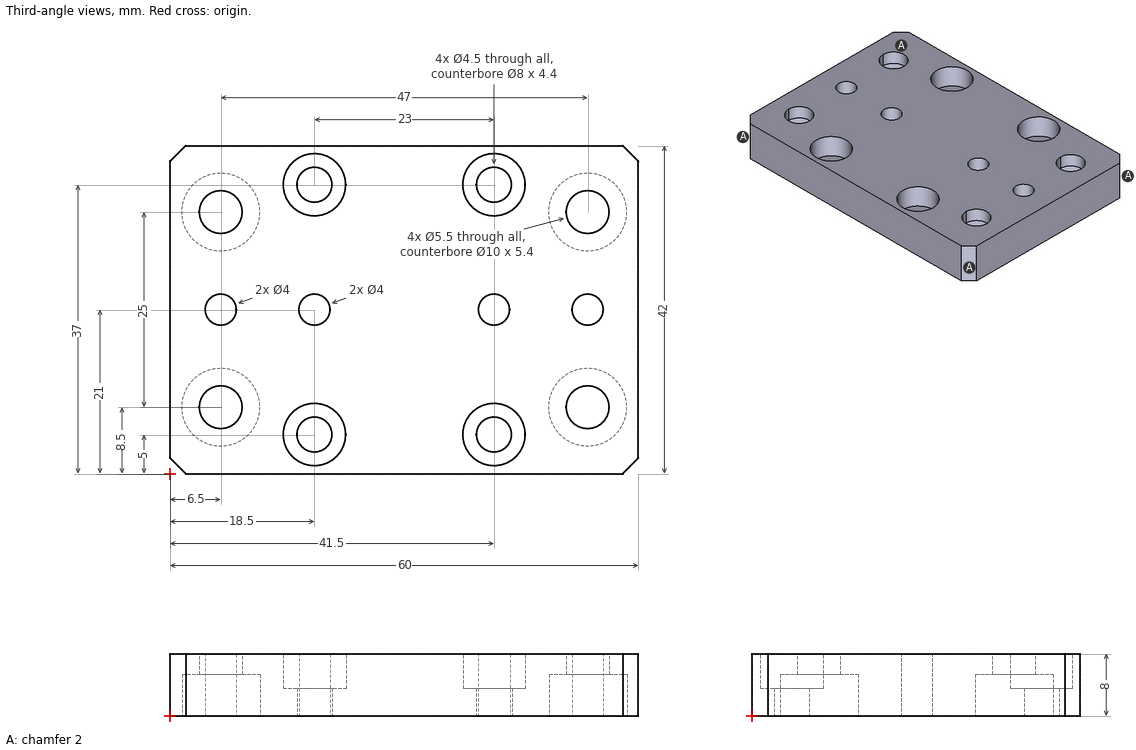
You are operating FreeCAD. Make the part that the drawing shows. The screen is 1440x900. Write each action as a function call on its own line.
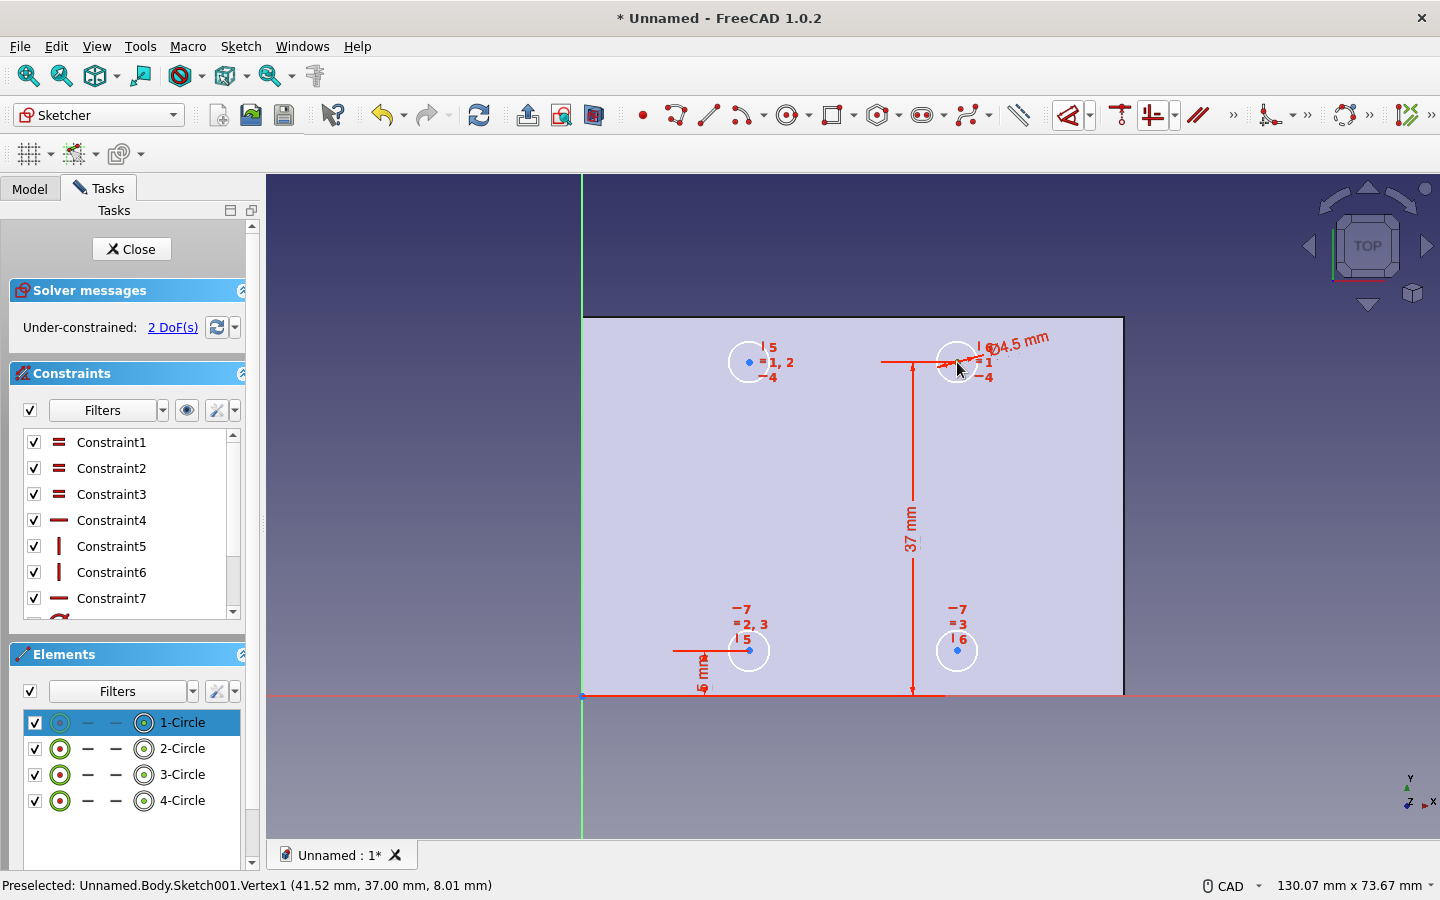
click(749, 362)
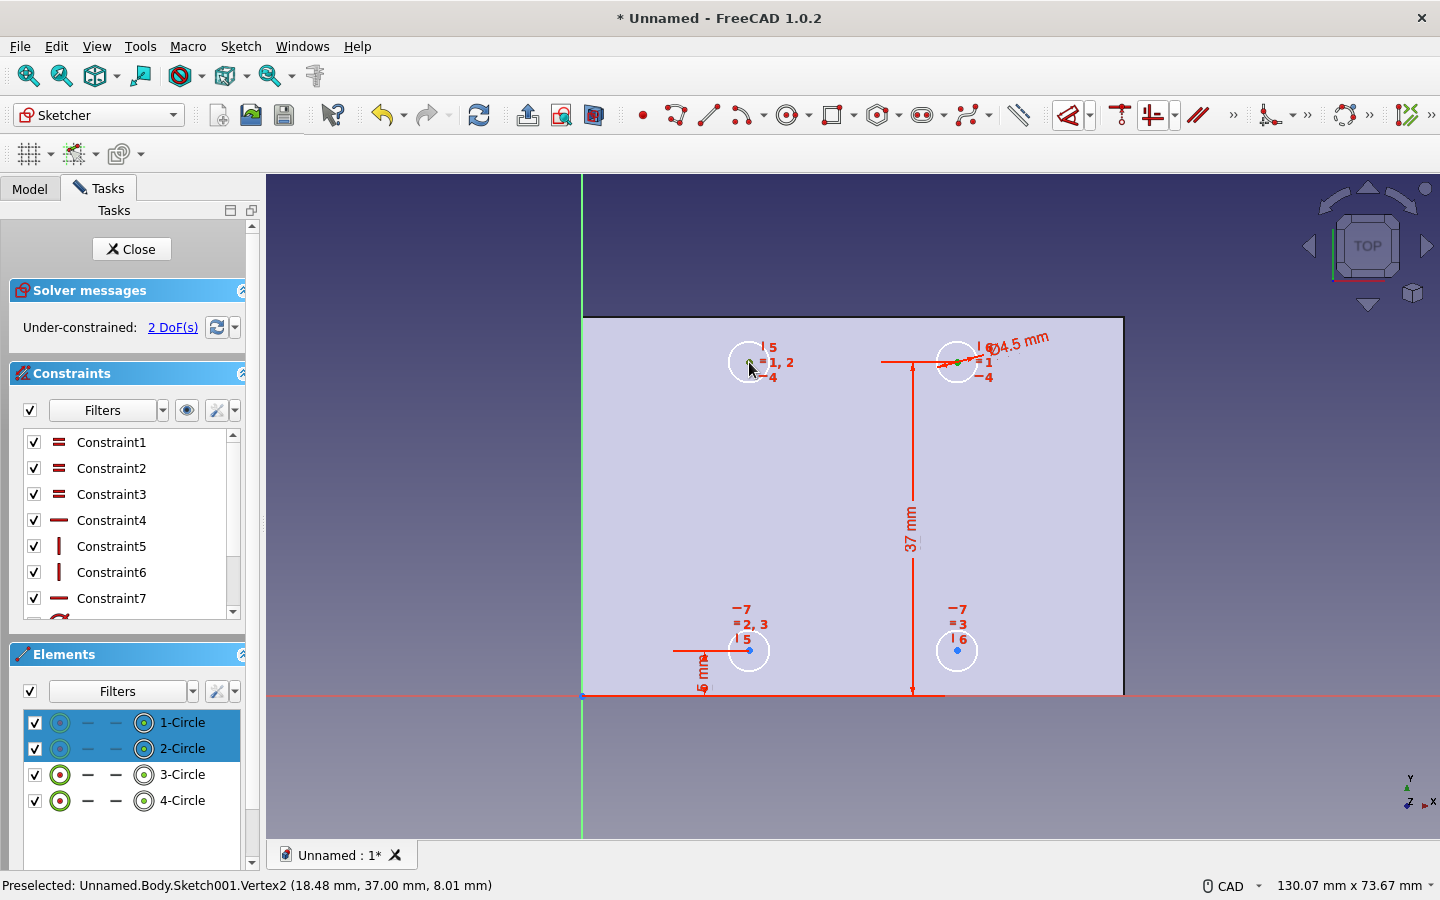
click(1090, 116)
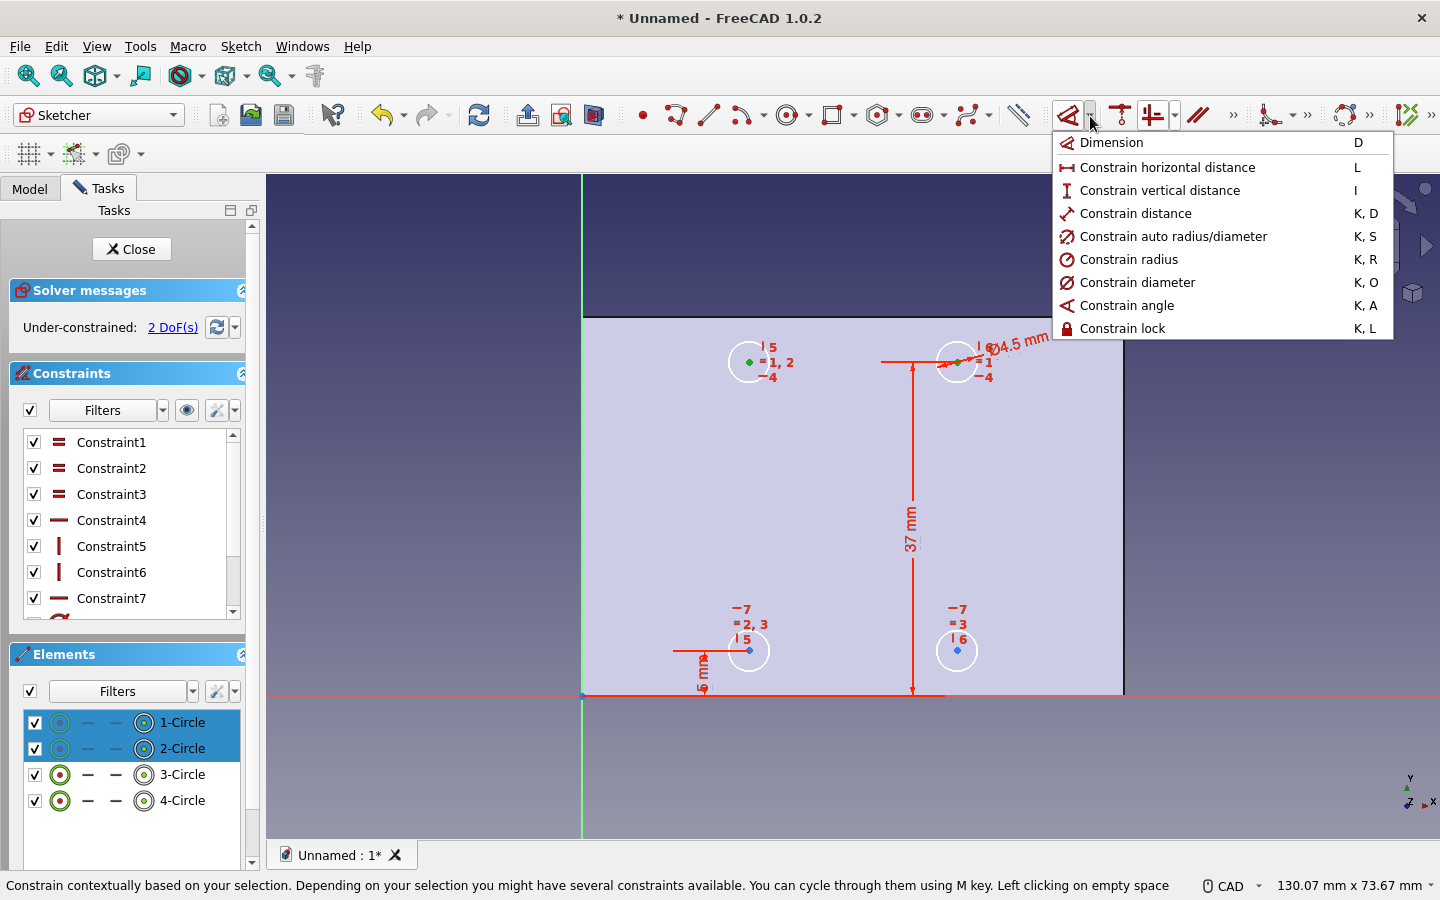
click(1223, 168)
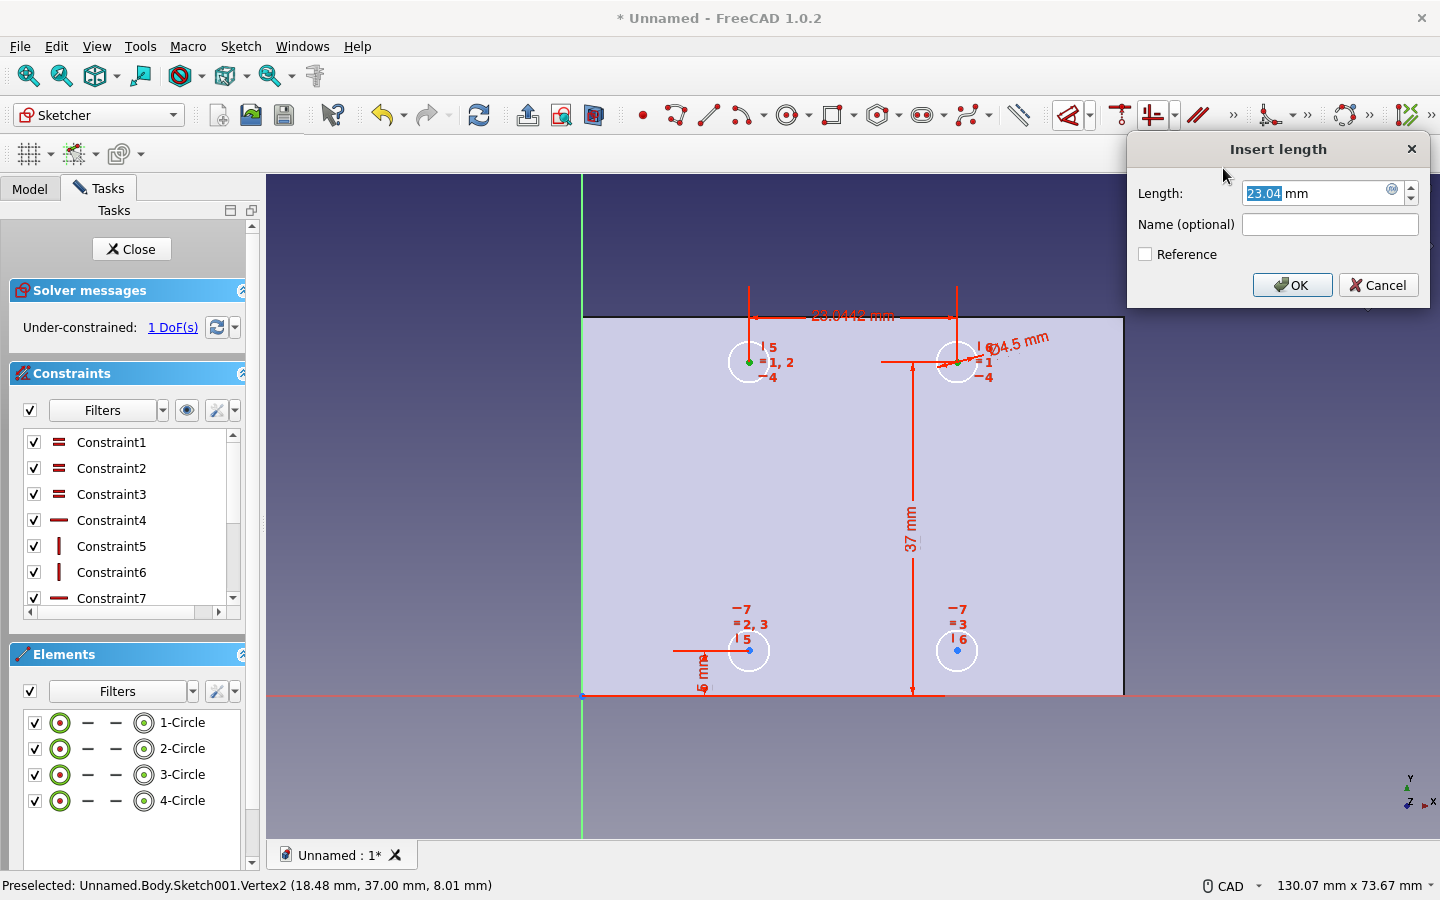
text(23)
key(Return)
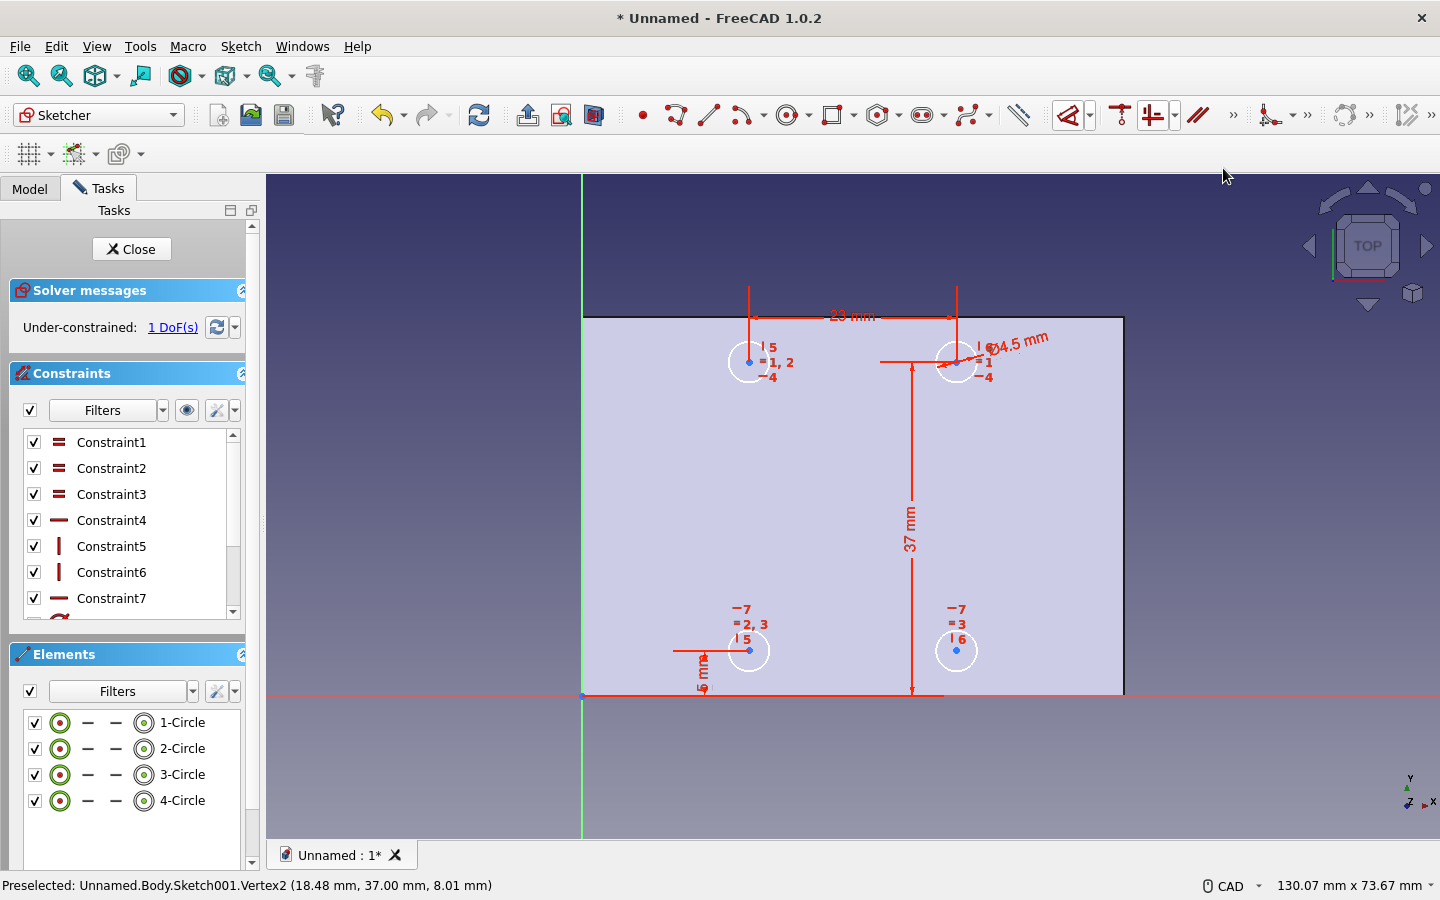
click(957, 362)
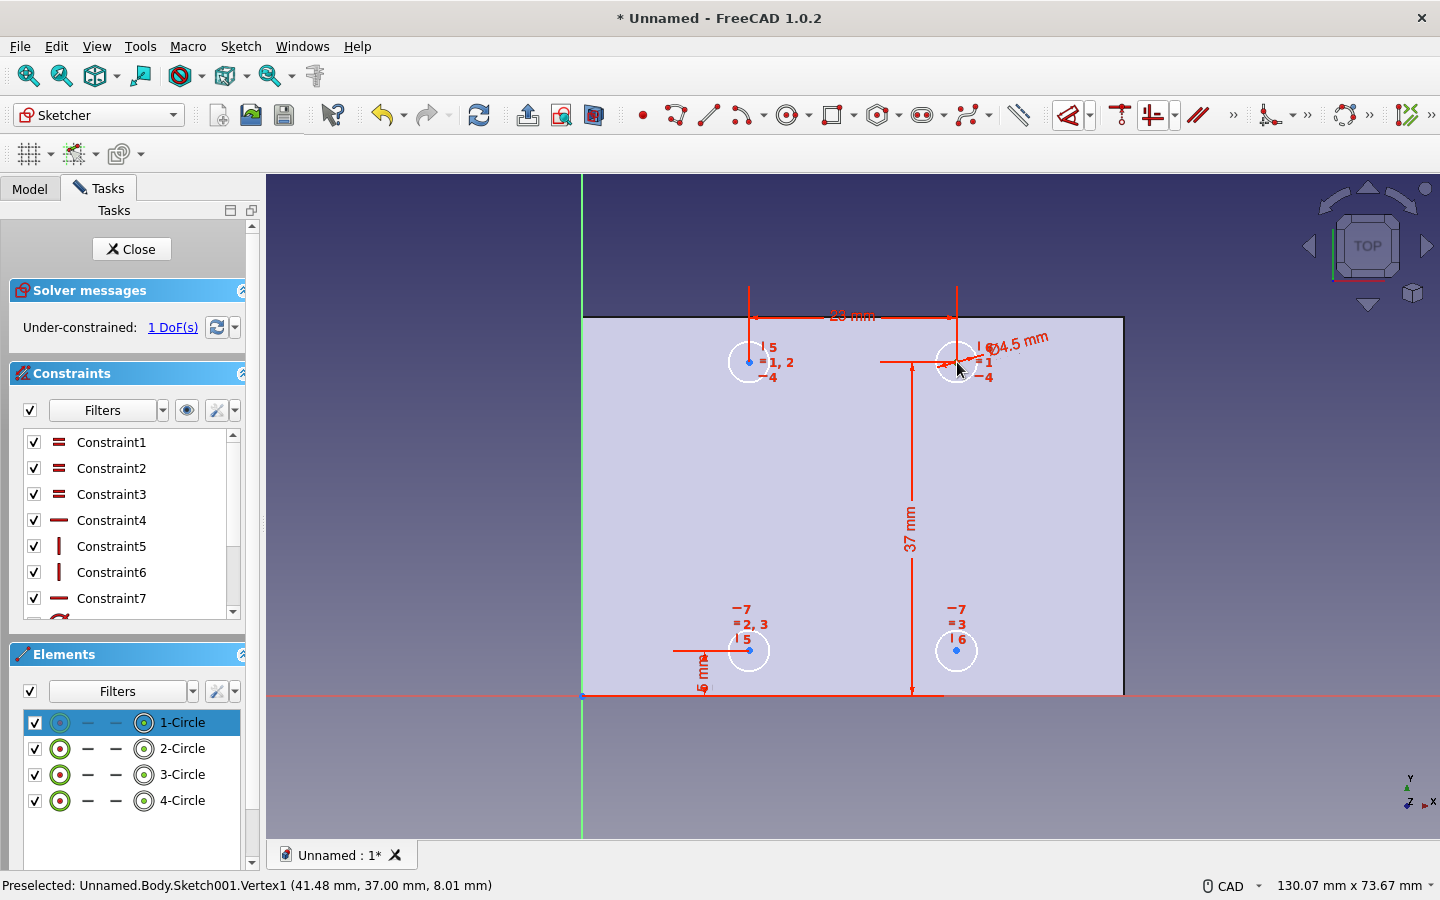
click(1090, 116)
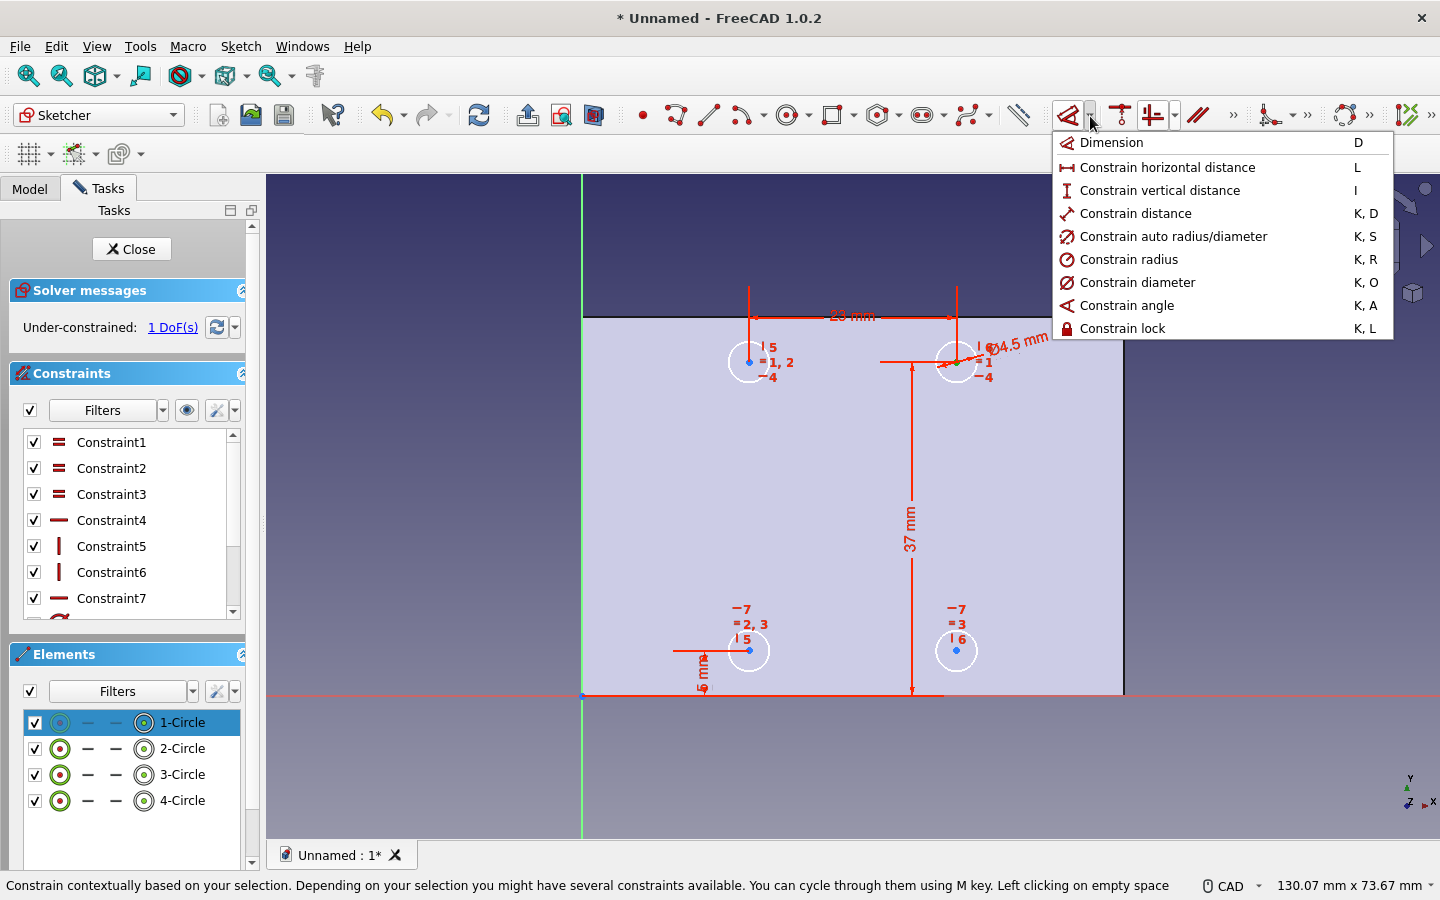
click(1223, 168)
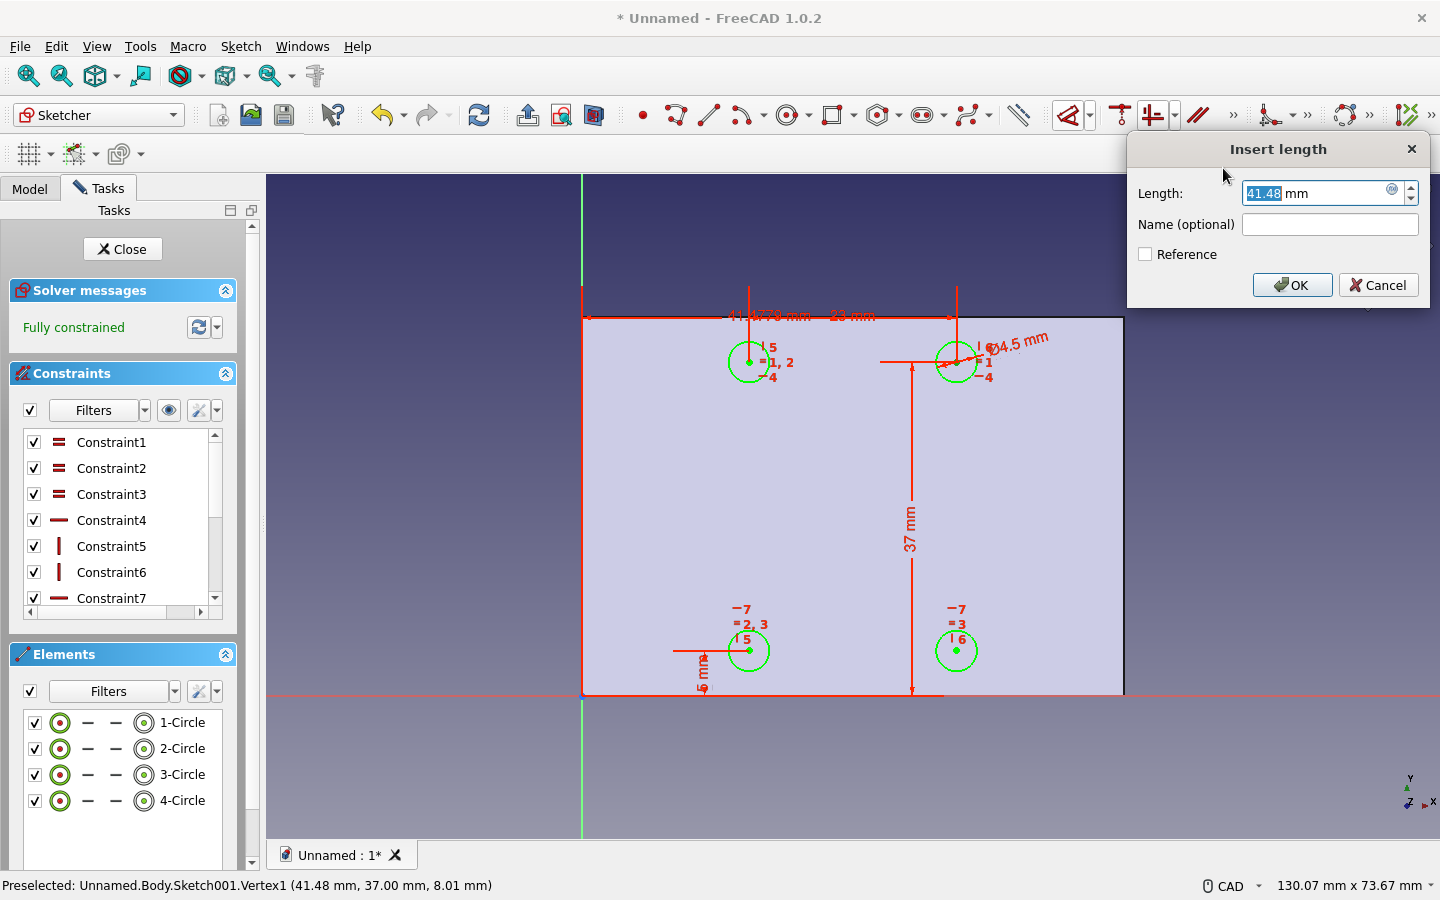
text(41.5)
key(Return)